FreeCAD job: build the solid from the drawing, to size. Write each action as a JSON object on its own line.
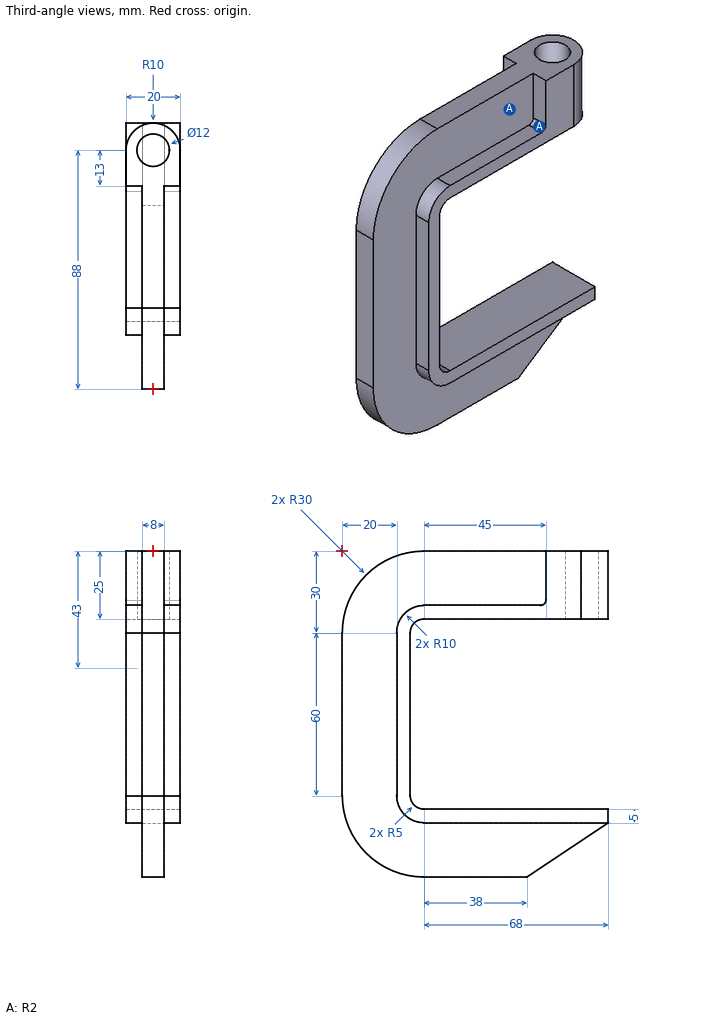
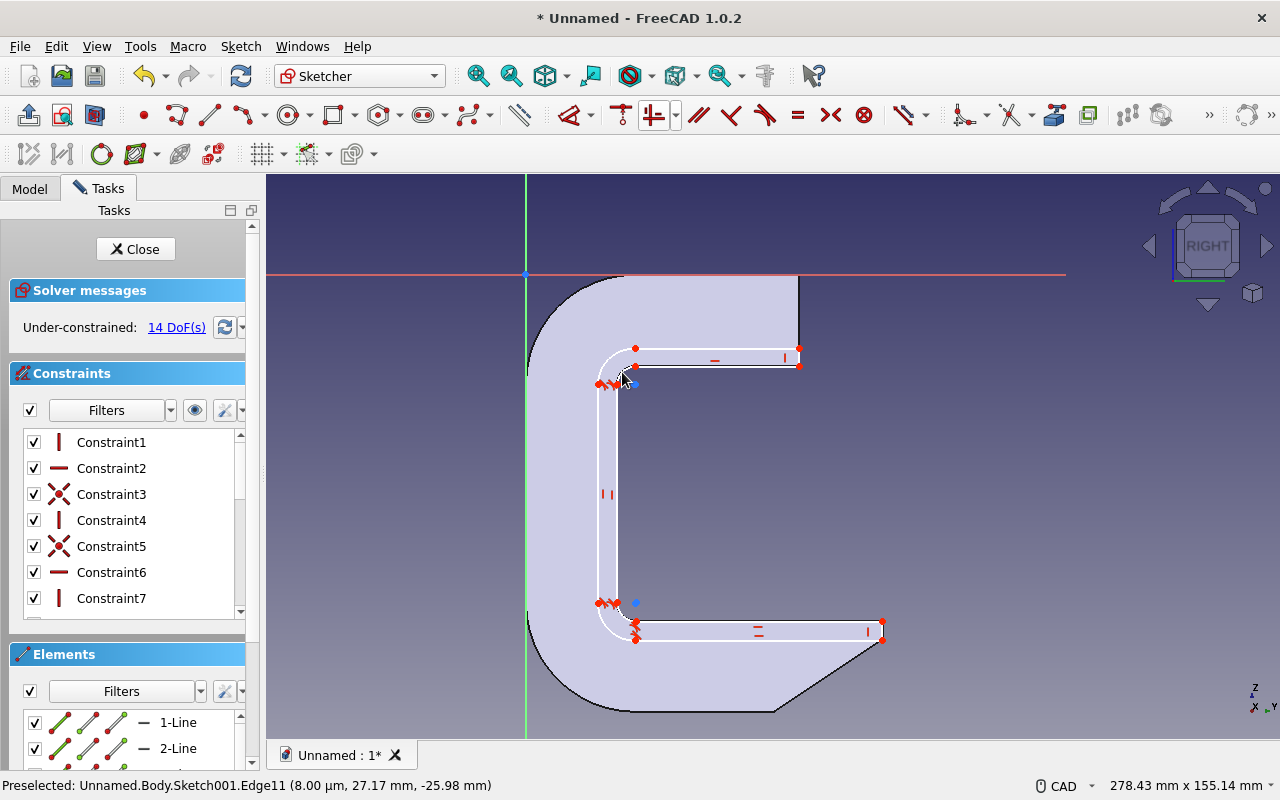
{"action": "left_click", "coordinate": [685, 367]}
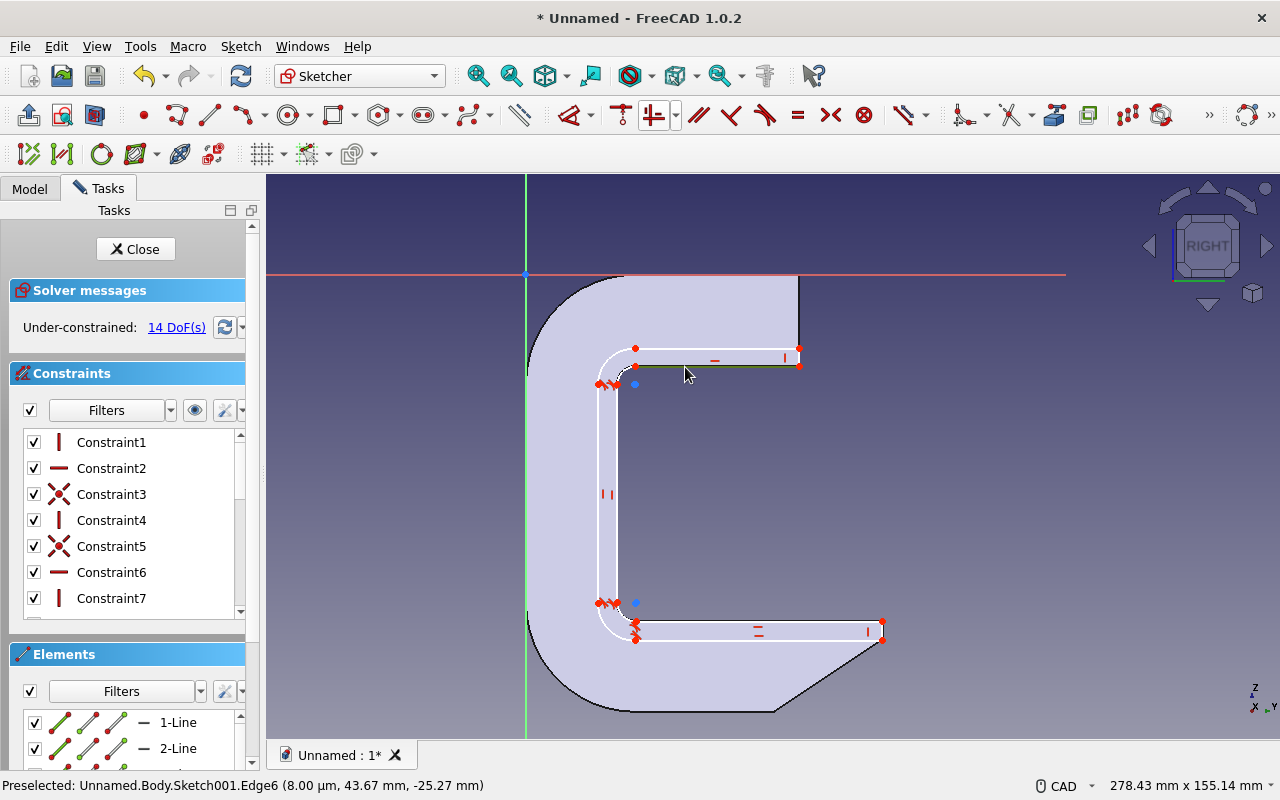
{"action": "left_click", "coordinate": [623, 372]}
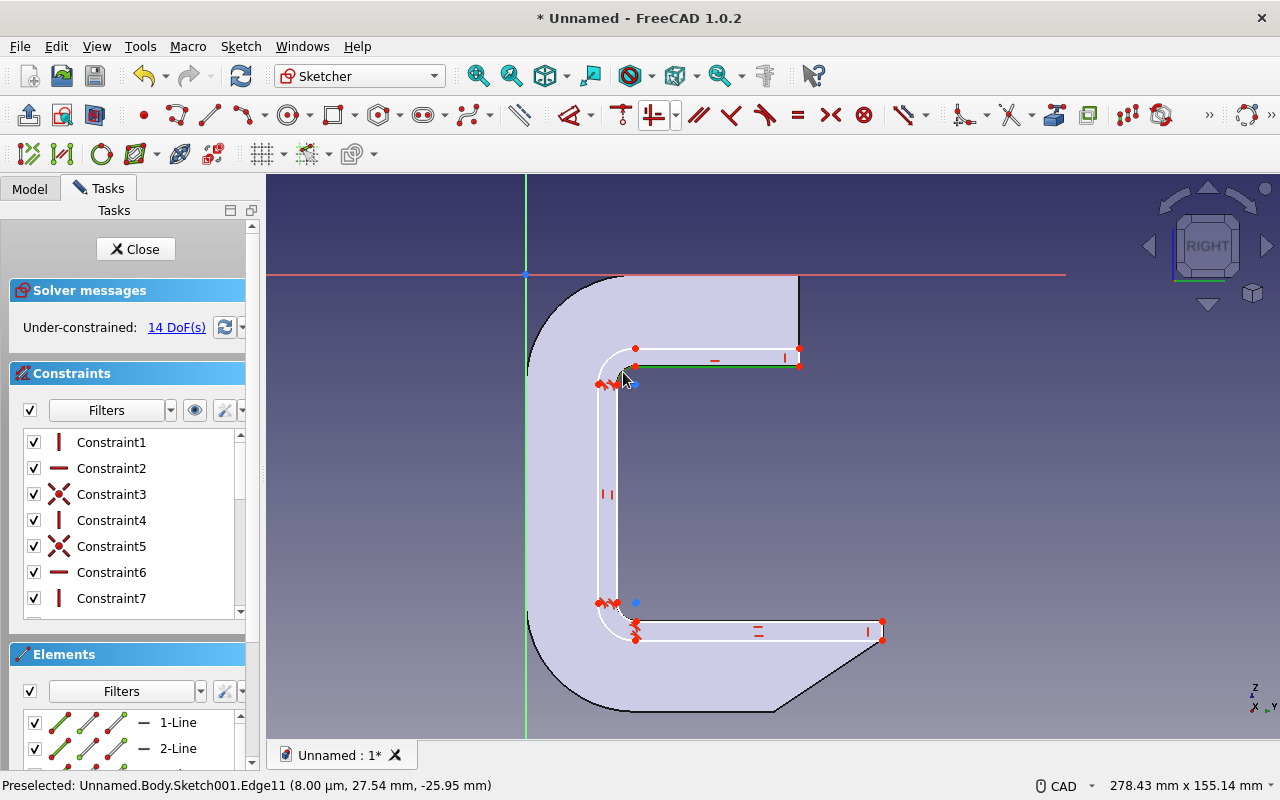
{"action": "key", "text": "t"}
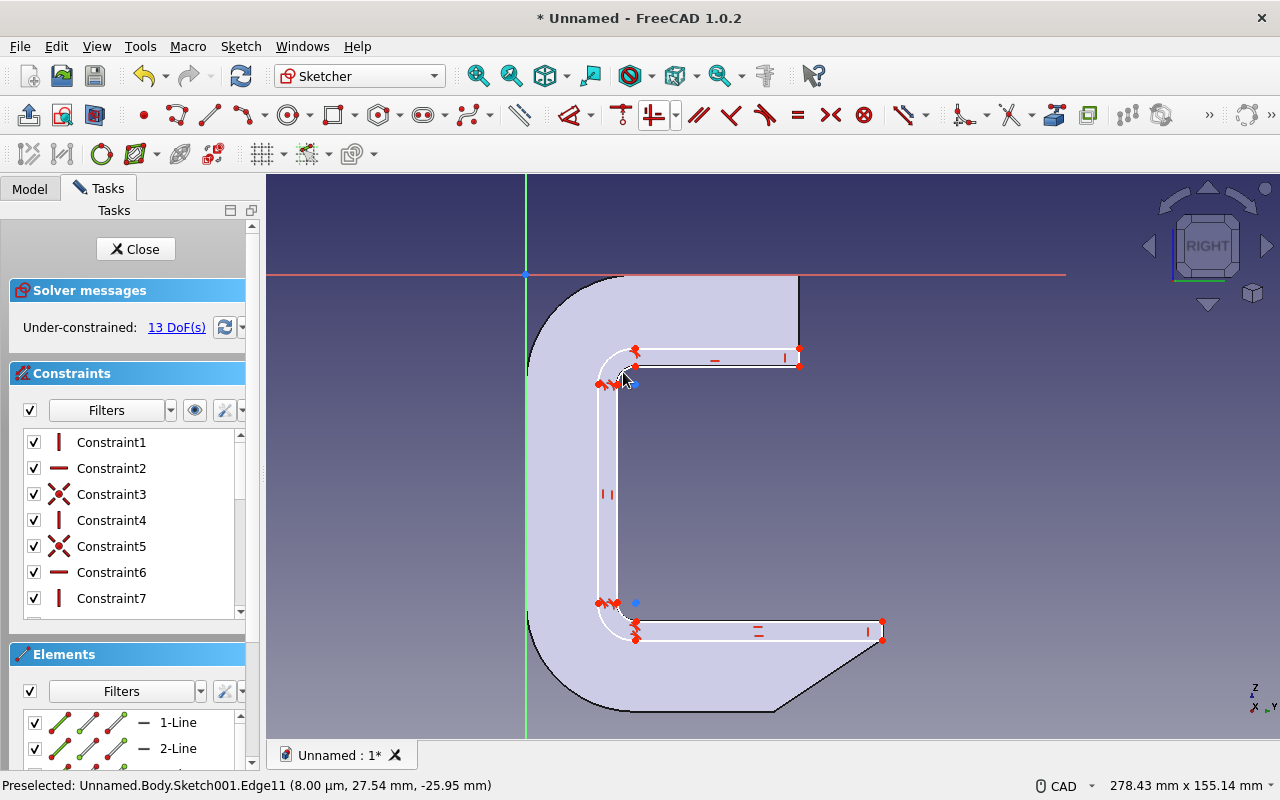
{"action": "left_click", "coordinate": [750, 349]}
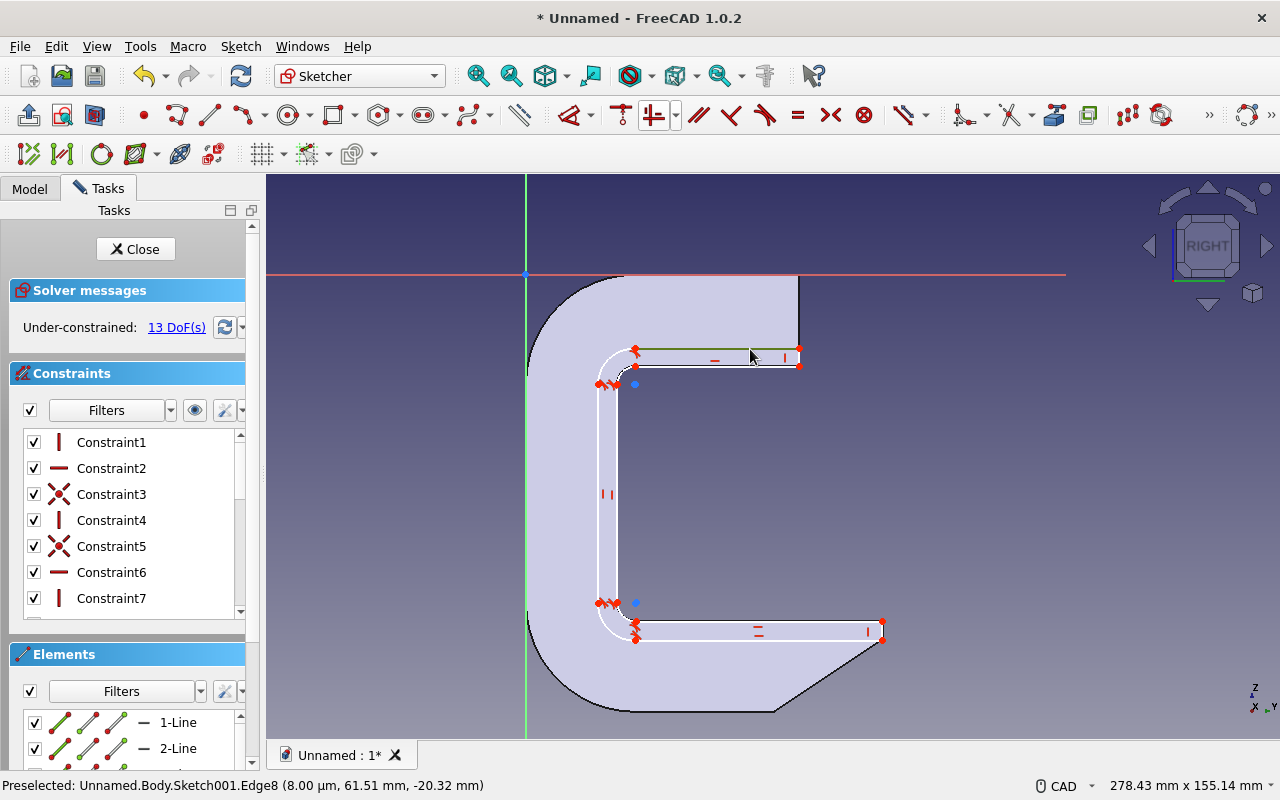
{"action": "left_click", "coordinate": [619, 352]}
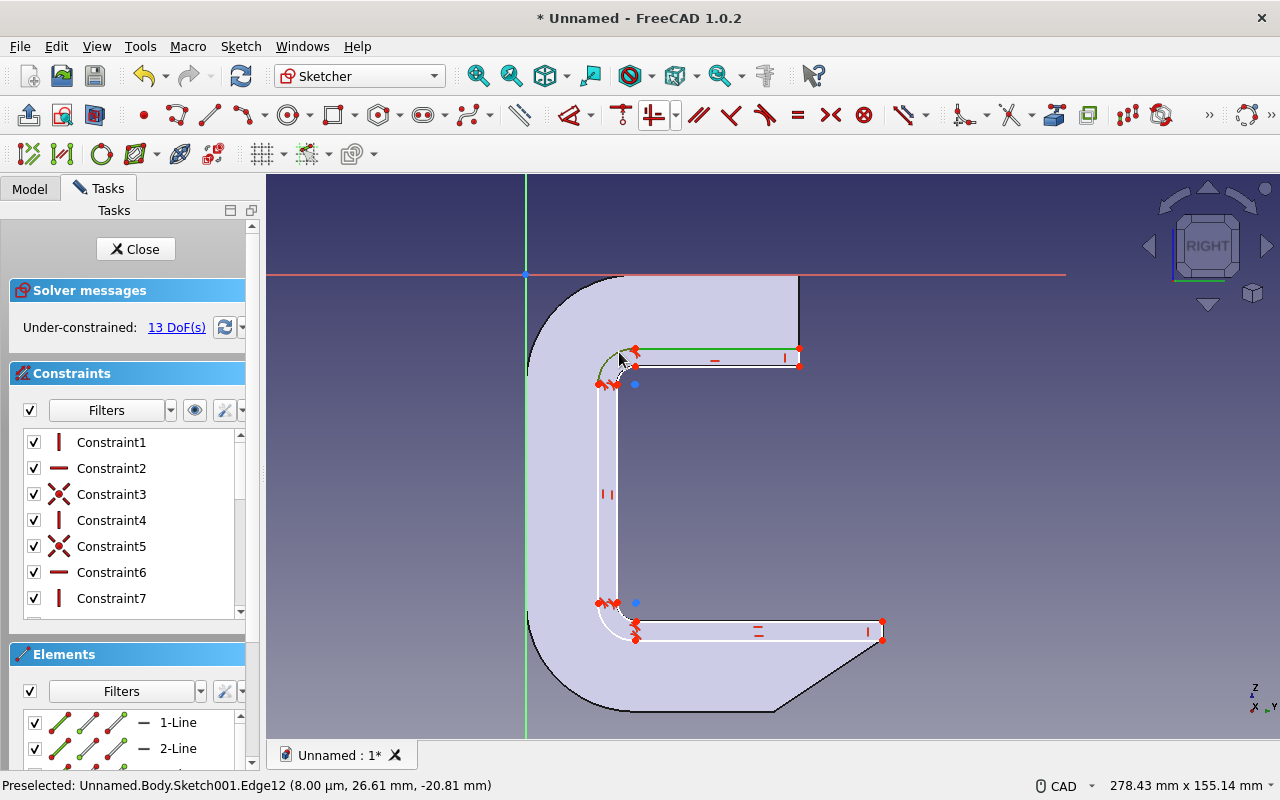
{"action": "key", "text": "t"}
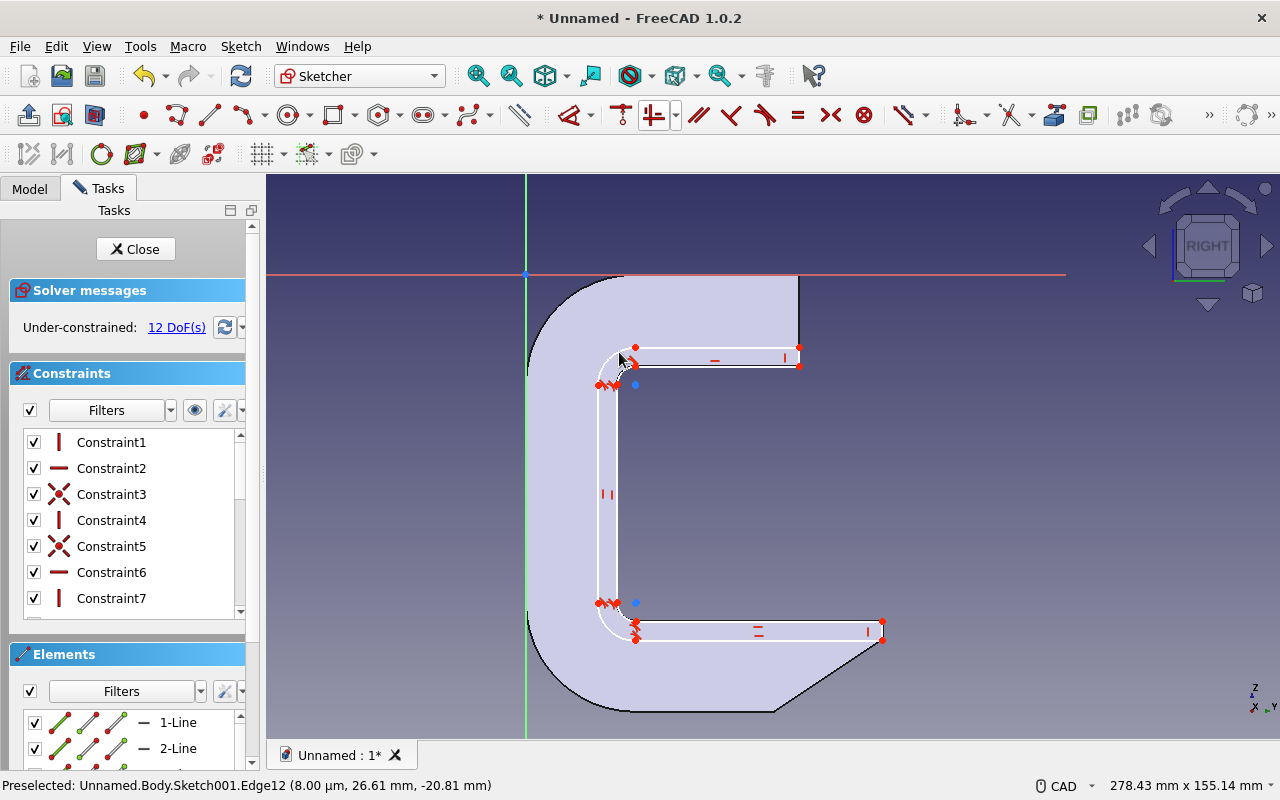
{"action": "left_click", "coordinate": [602, 620]}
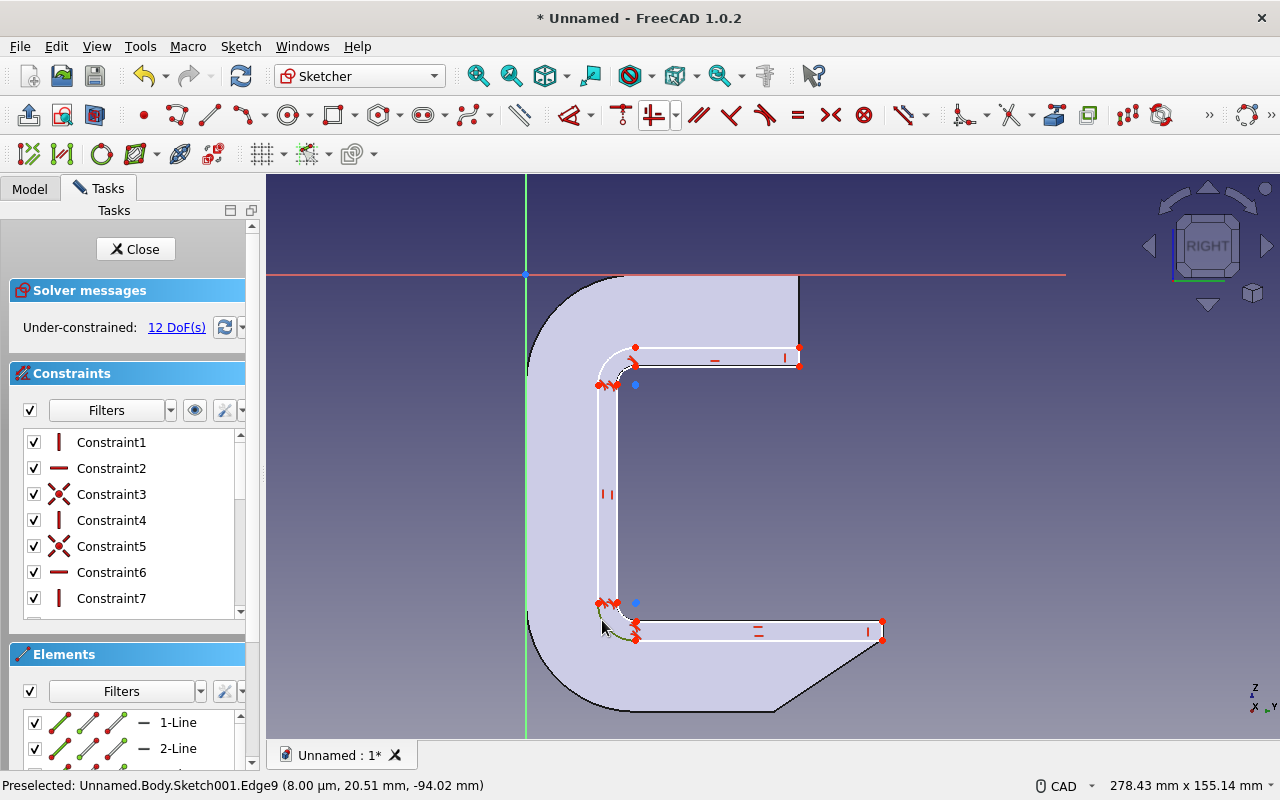
{"action": "left_click", "coordinate": [623, 616]}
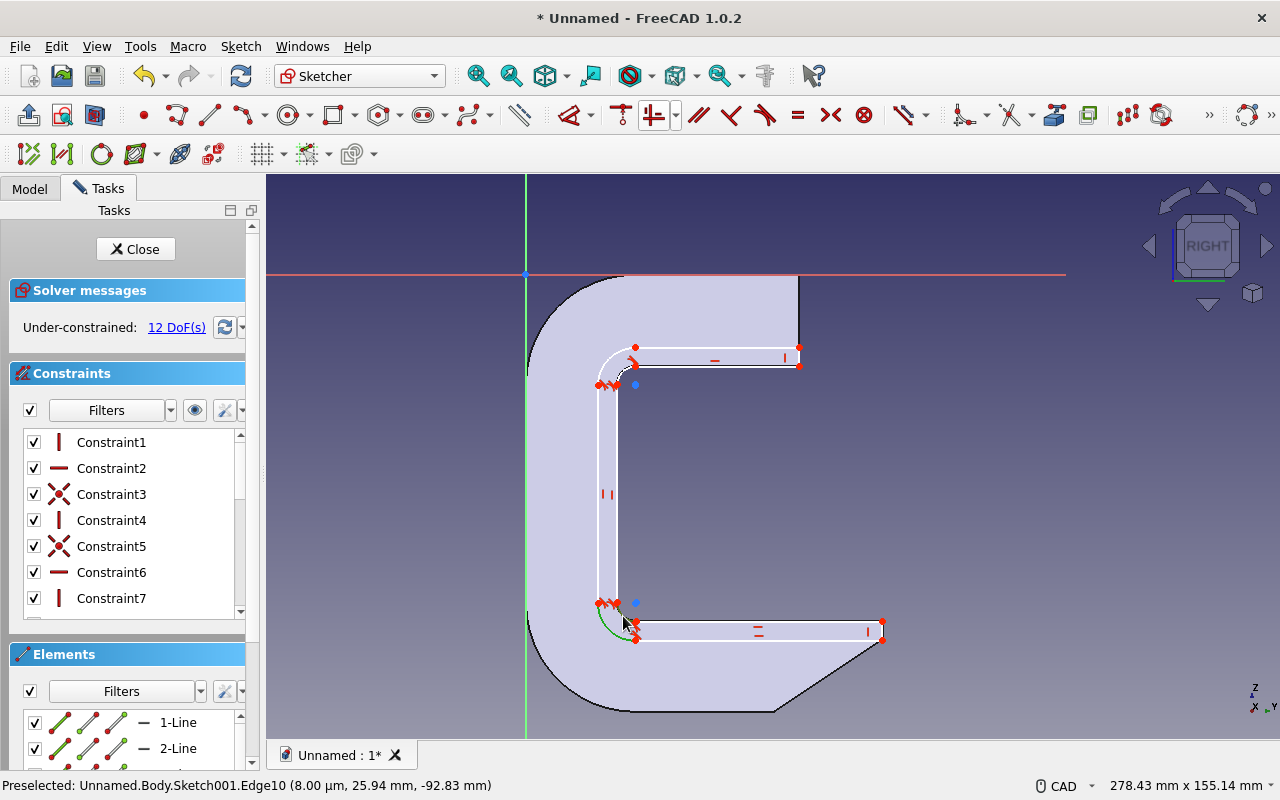
{"action": "left_click", "coordinate": [621, 116]}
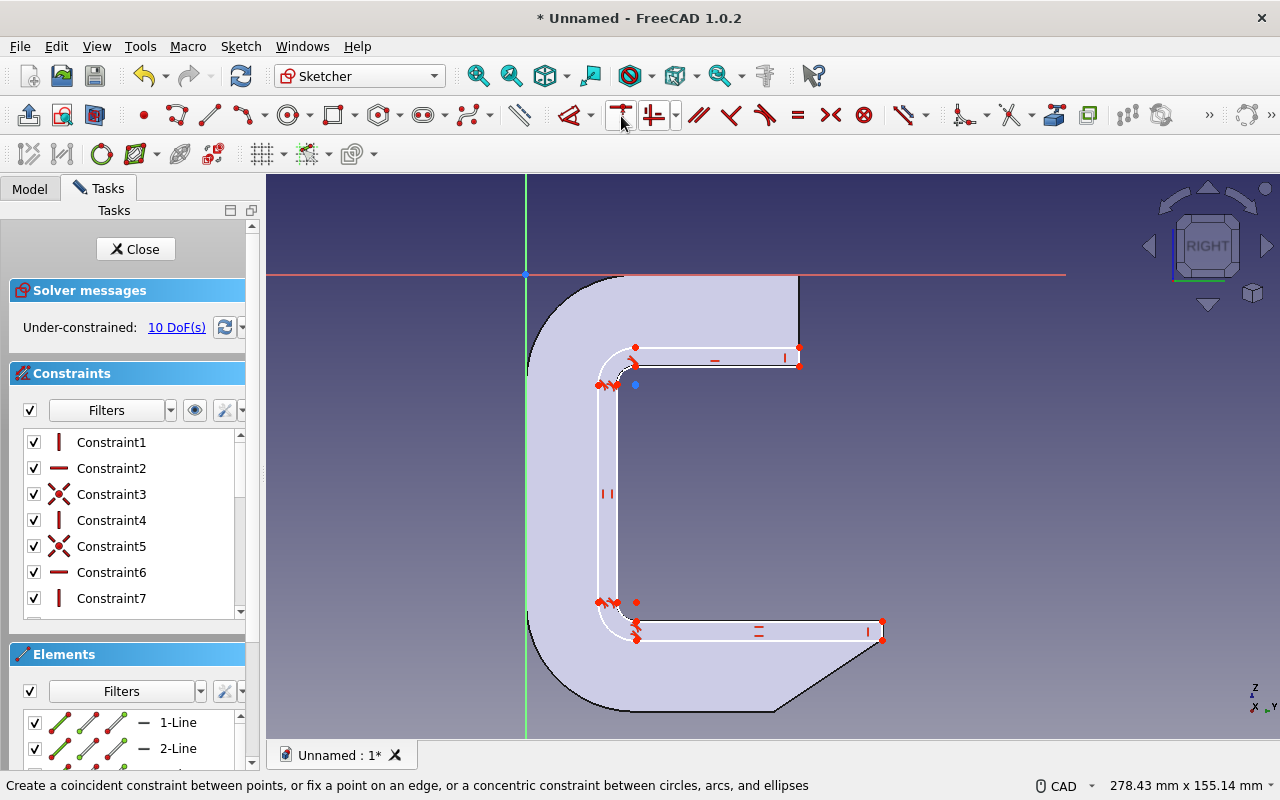
{"action": "left_click", "coordinate": [623, 372]}